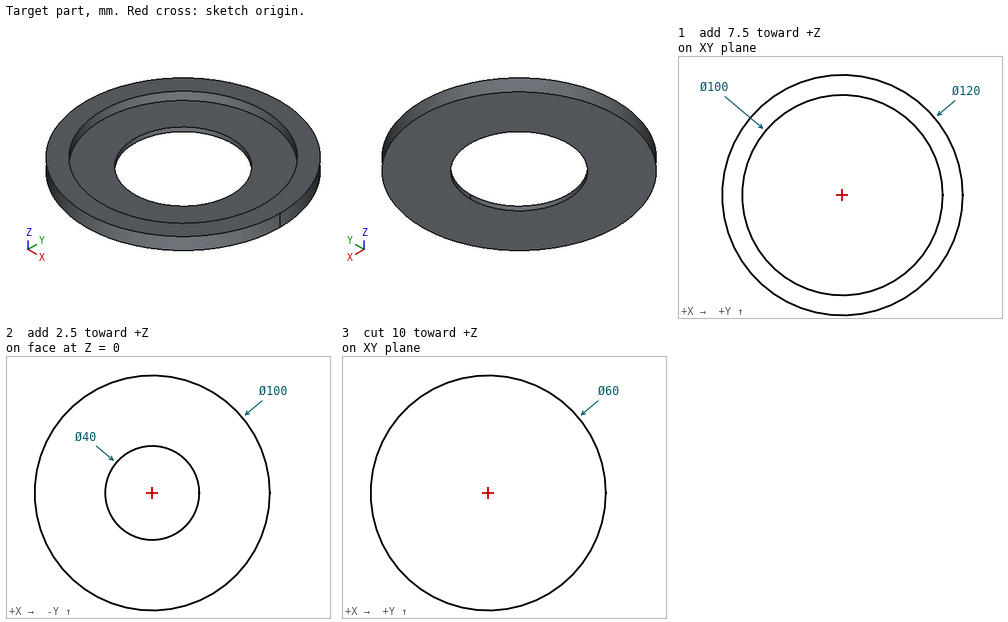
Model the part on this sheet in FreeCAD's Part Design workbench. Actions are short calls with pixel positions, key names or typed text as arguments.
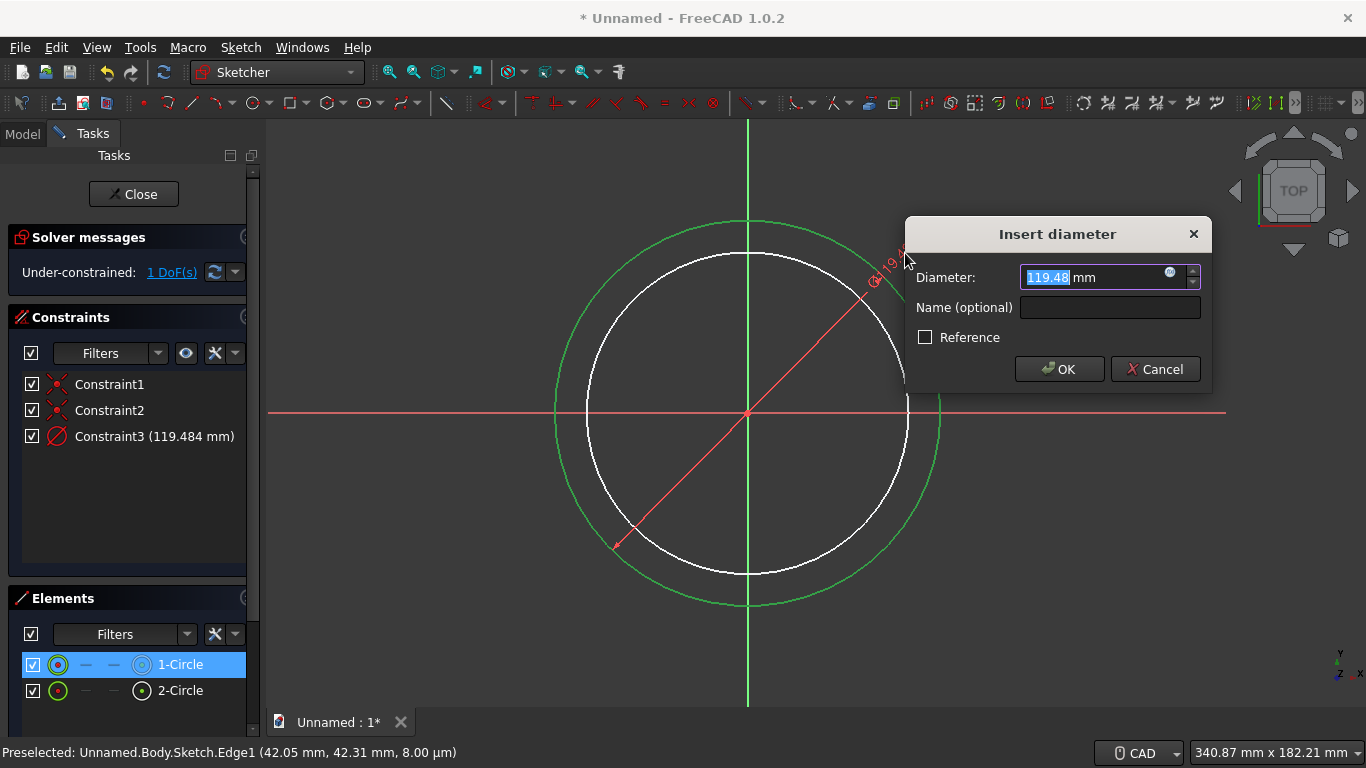
text(120)
key(Return)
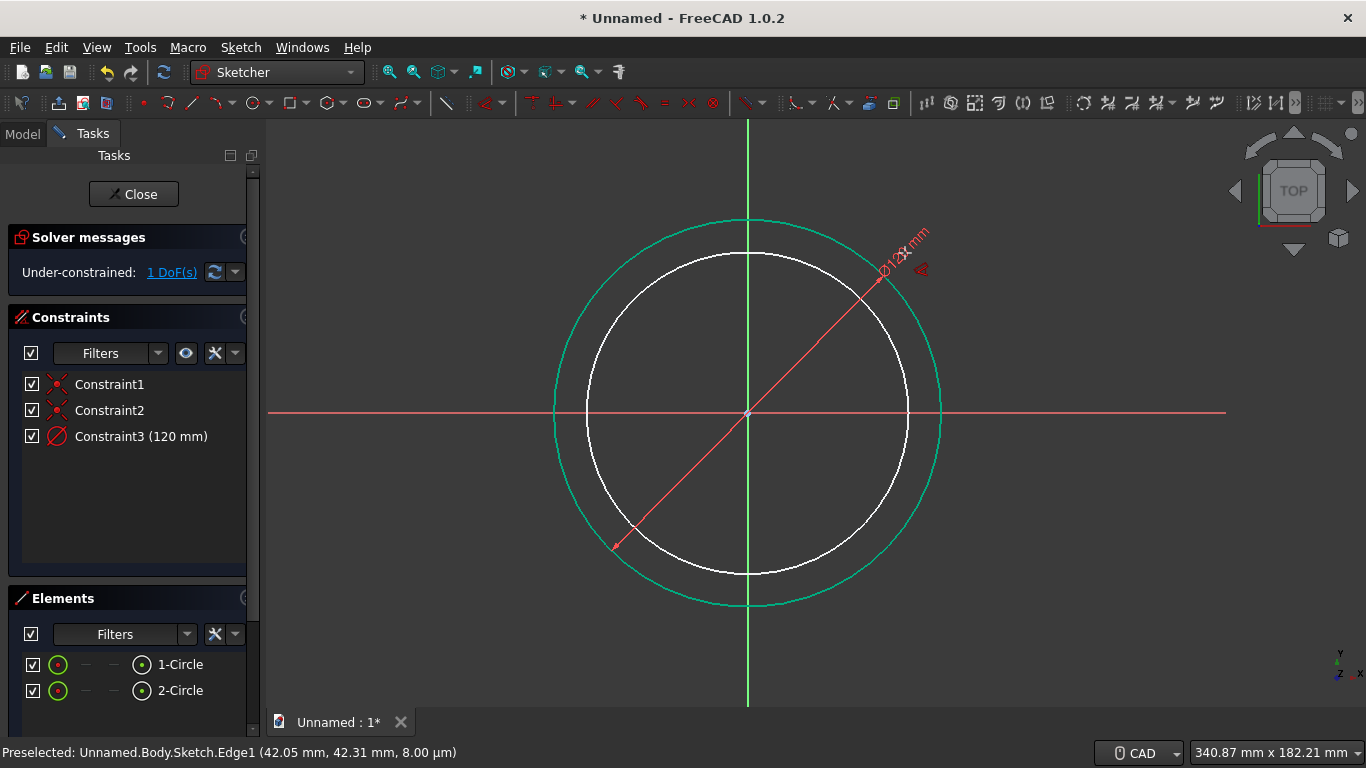
click(861, 299)
click(955, 352)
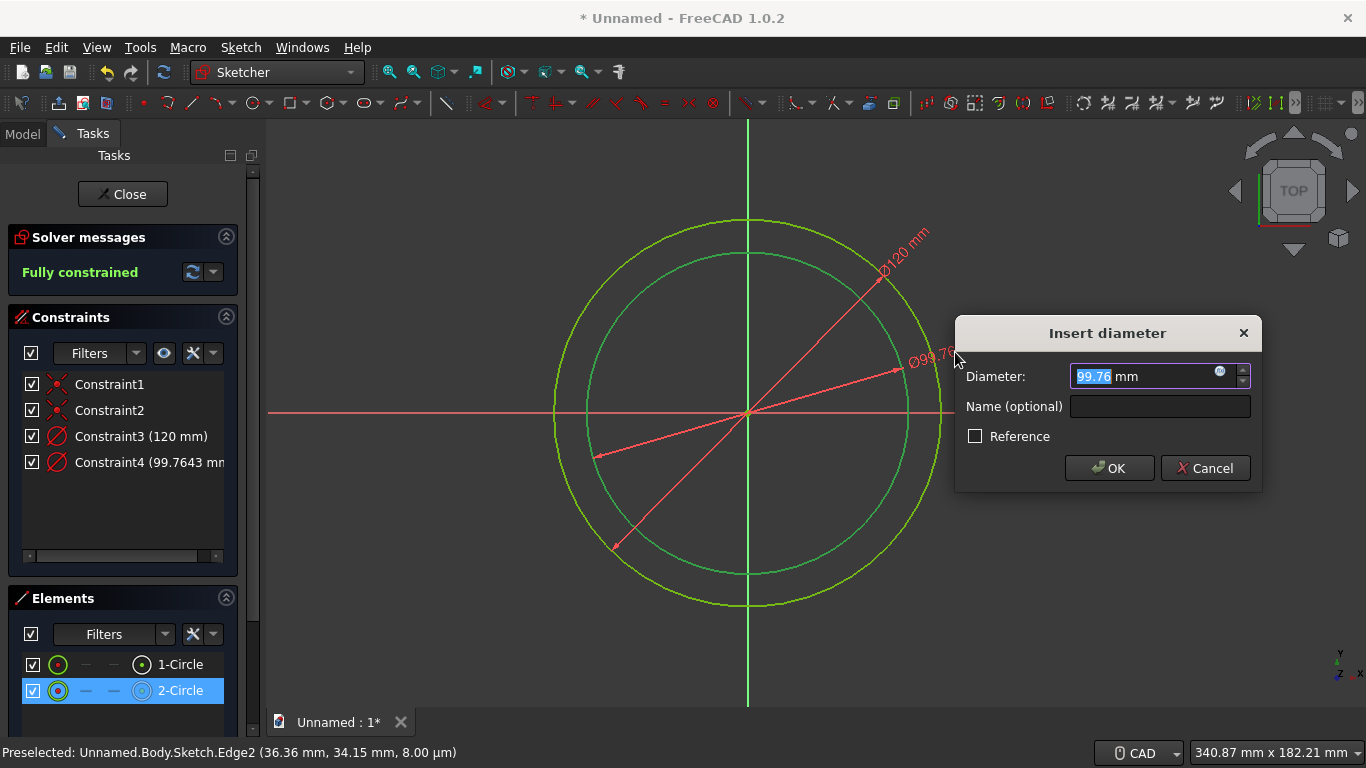
text(100)
key(Return)
key(Escape)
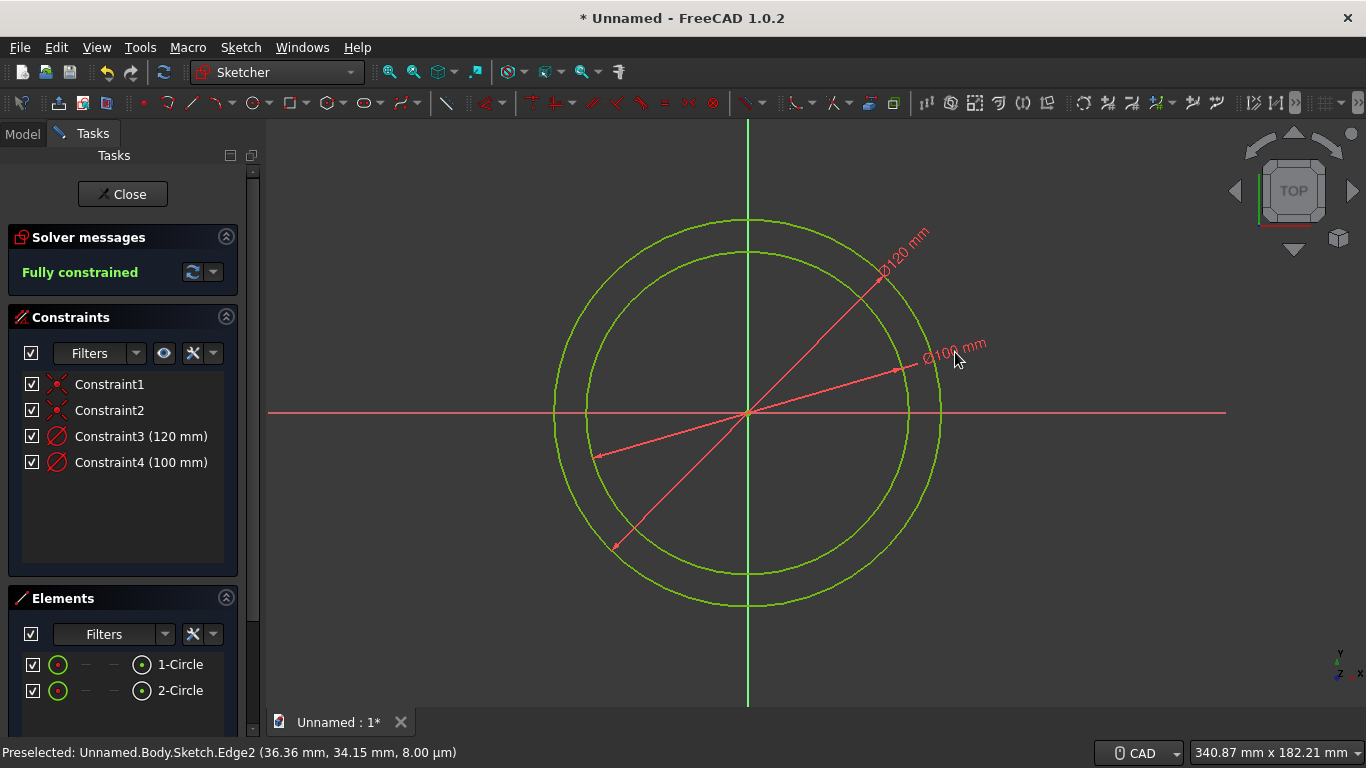
click(123, 194)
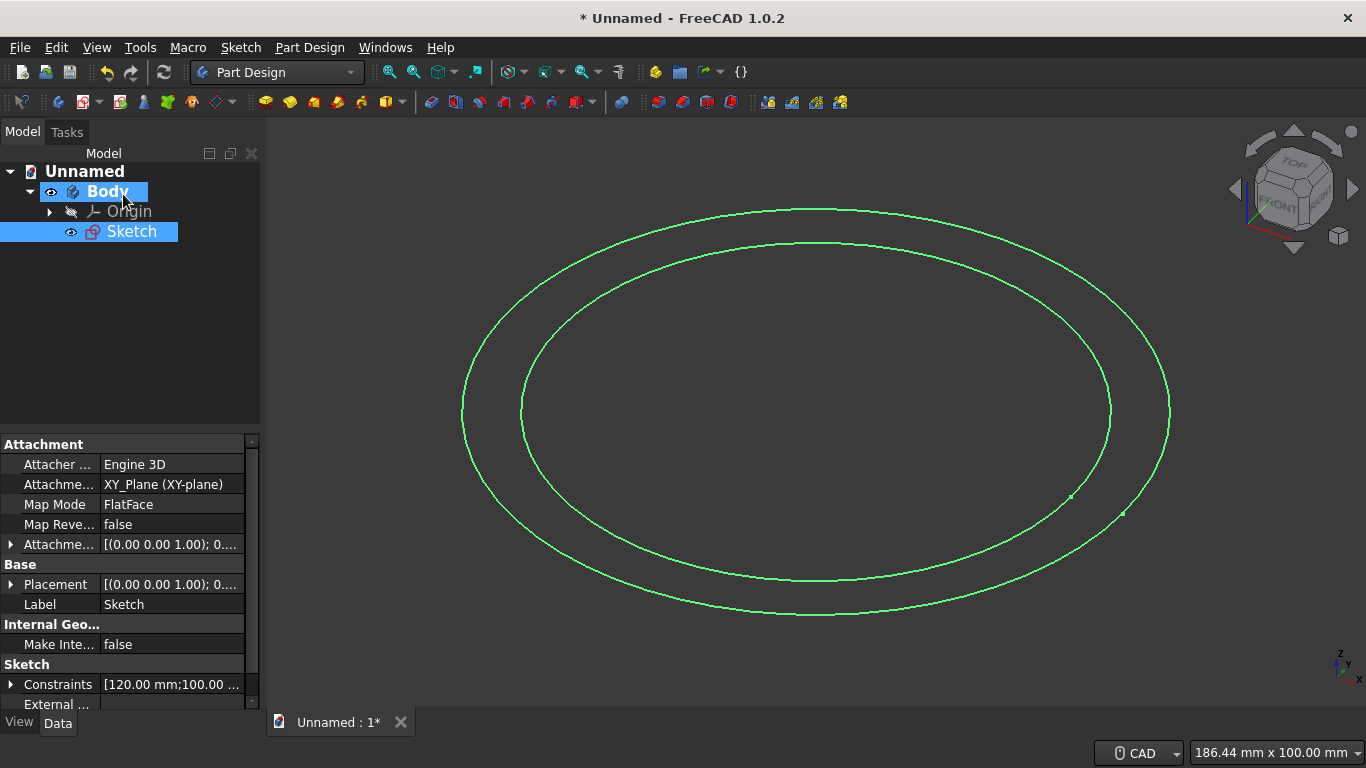
click(266, 102)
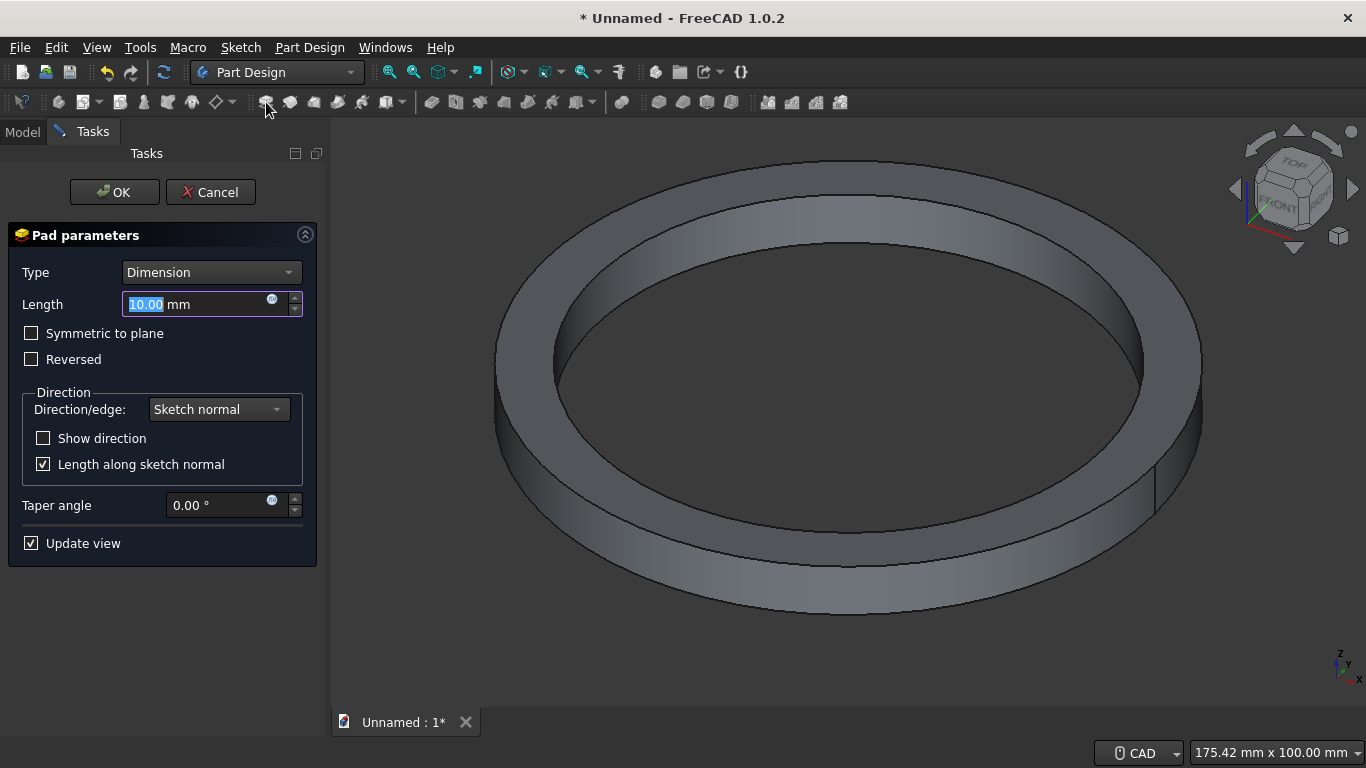
text(7.5)
key(Tab)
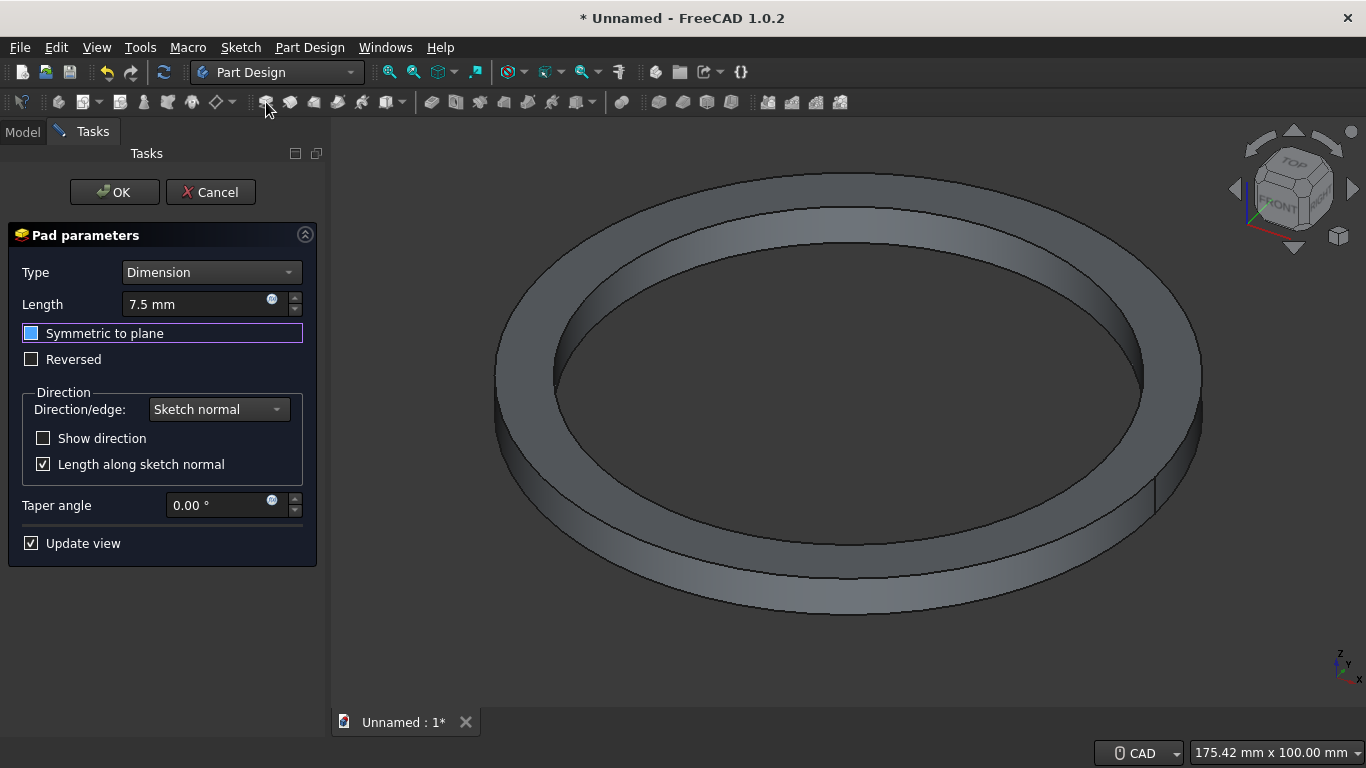
click(115, 192)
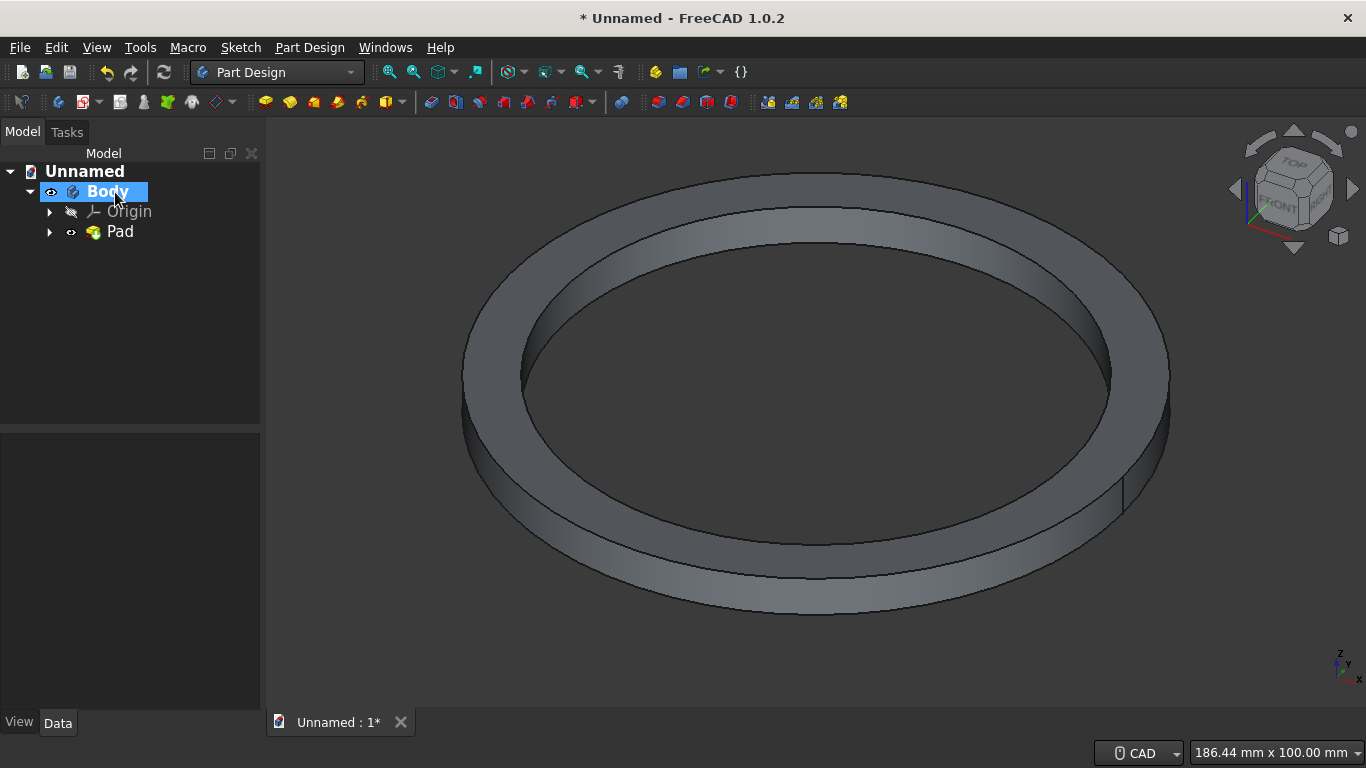
click(390, 72)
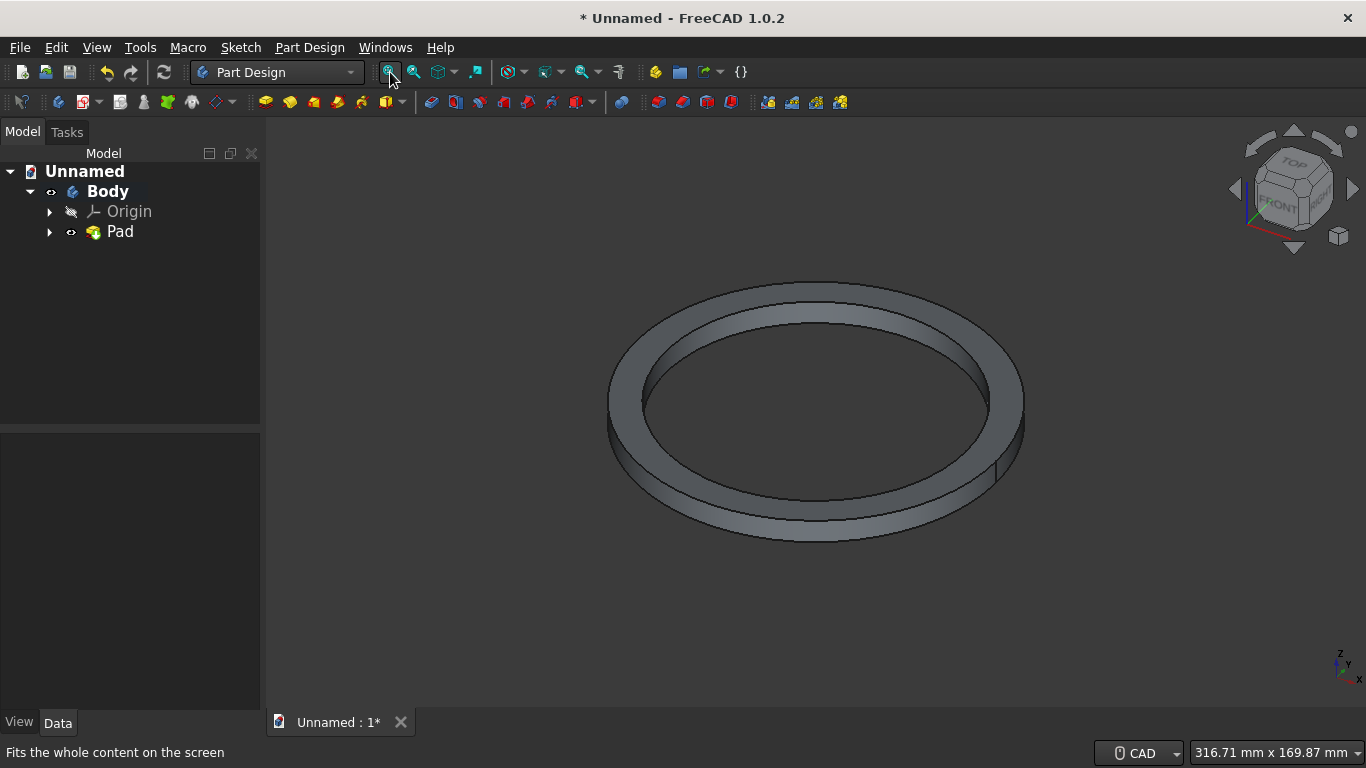
key(5)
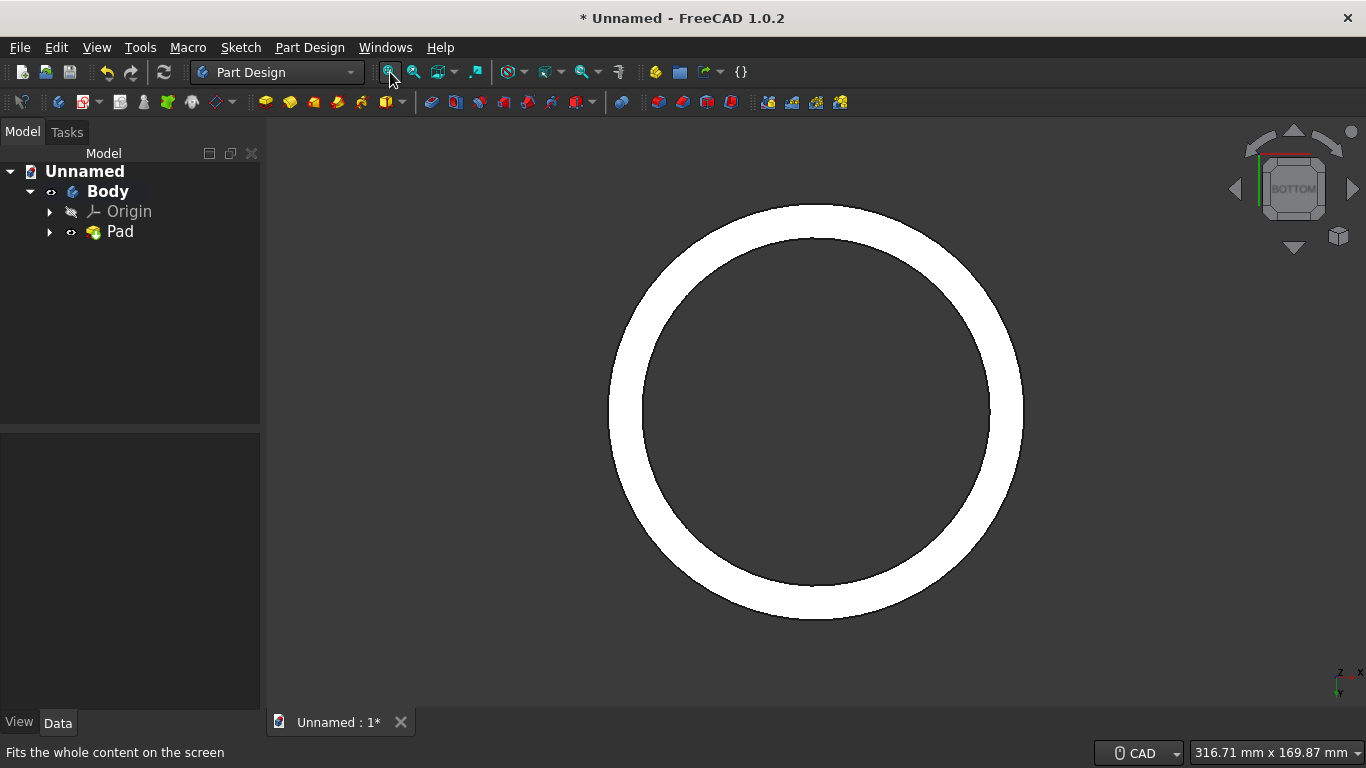
click(756, 590)